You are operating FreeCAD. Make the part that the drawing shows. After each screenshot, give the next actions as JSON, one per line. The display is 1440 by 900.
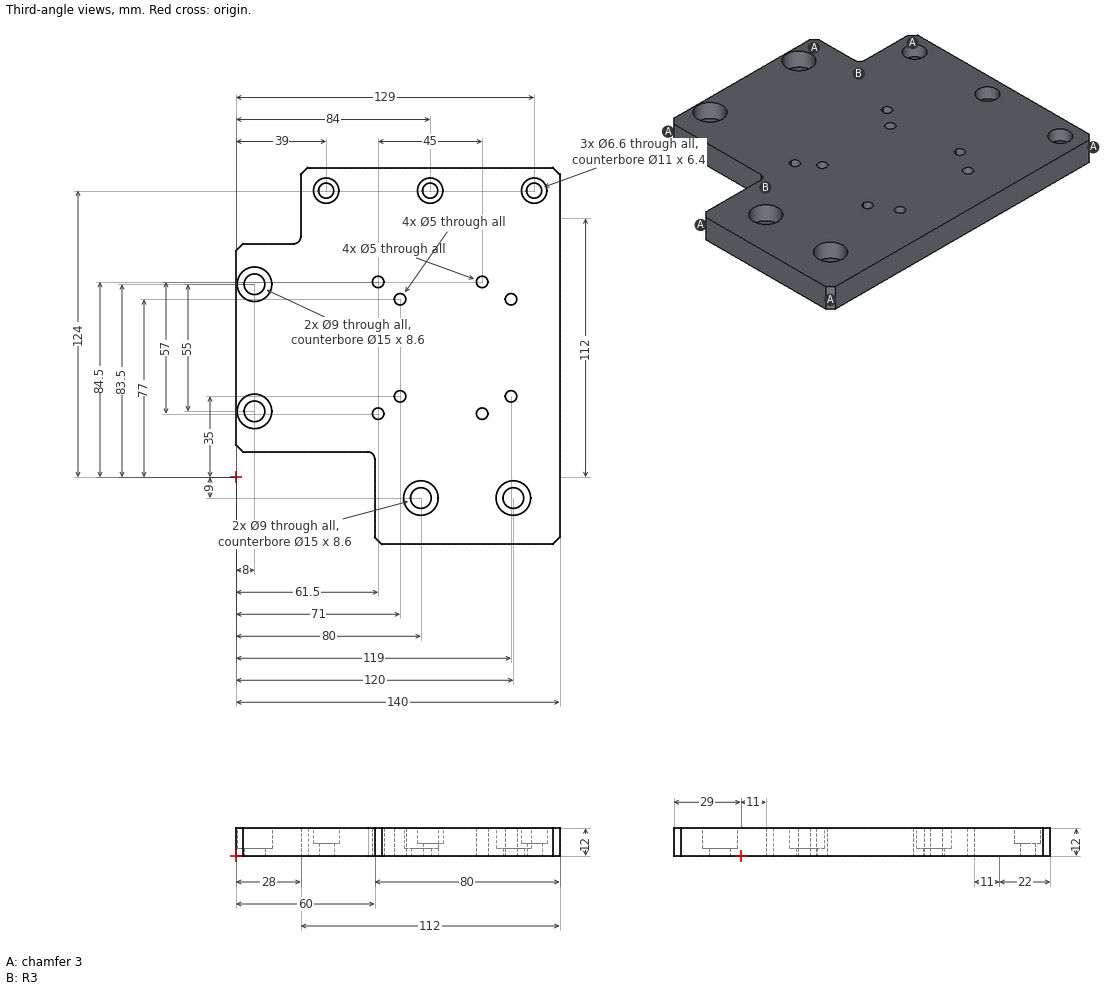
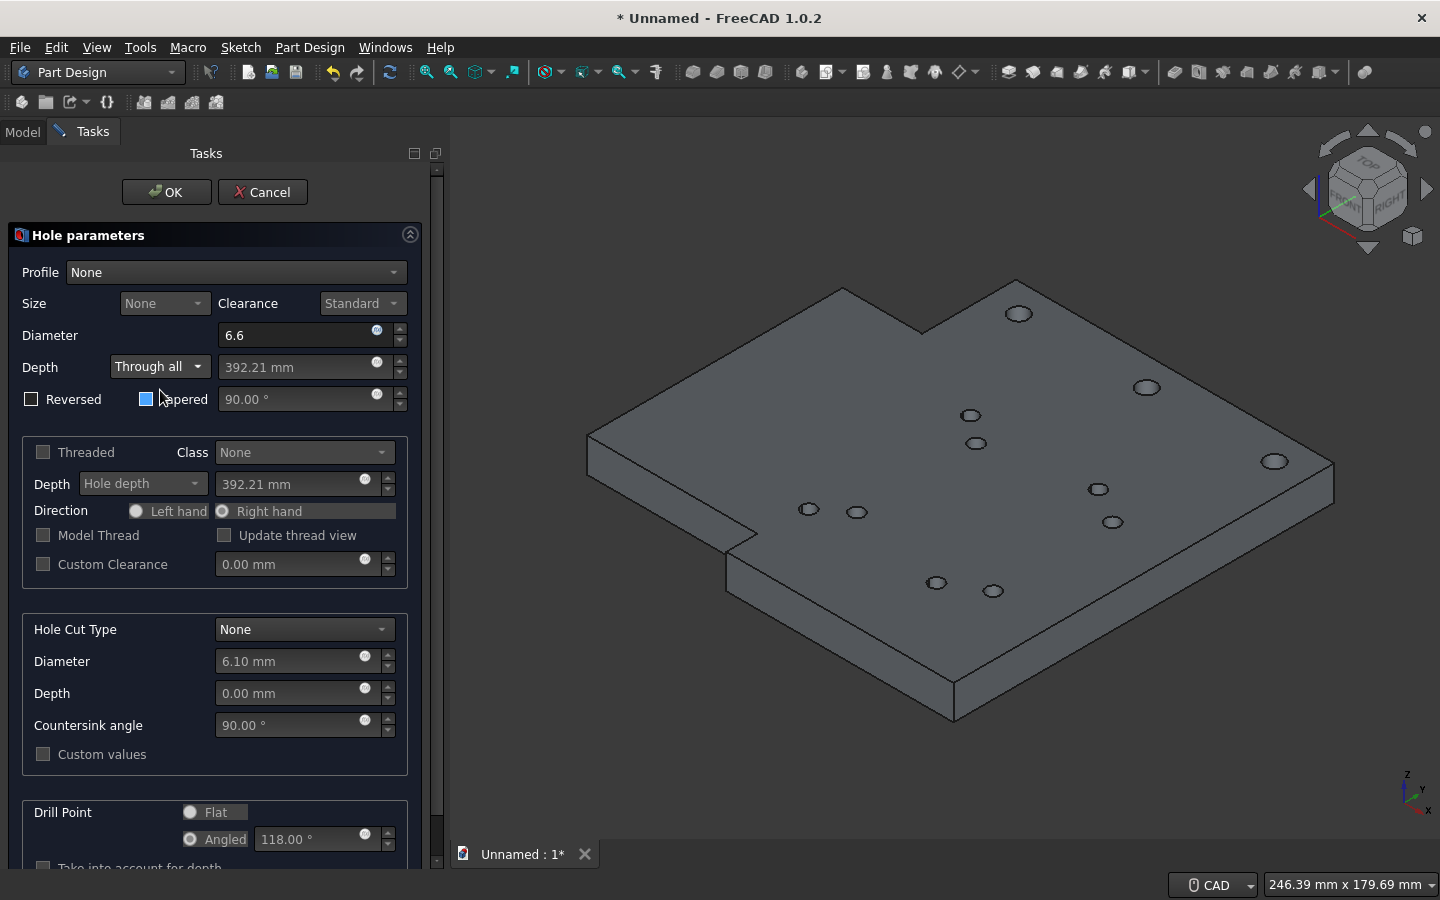
{"action": "left_click", "coordinate": [306, 630]}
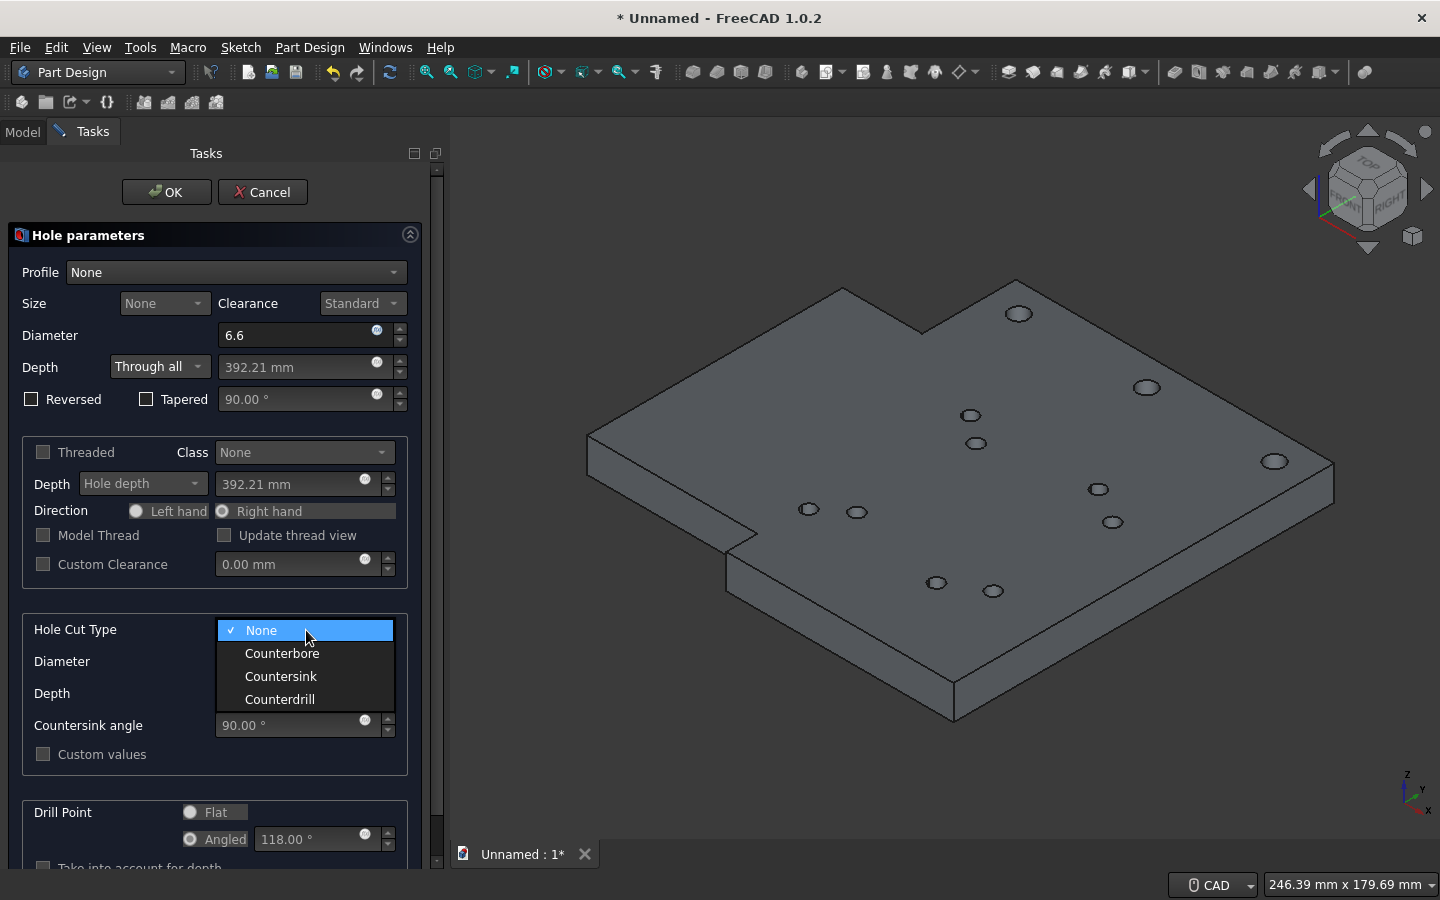
{"action": "left_click", "coordinate": [304, 654]}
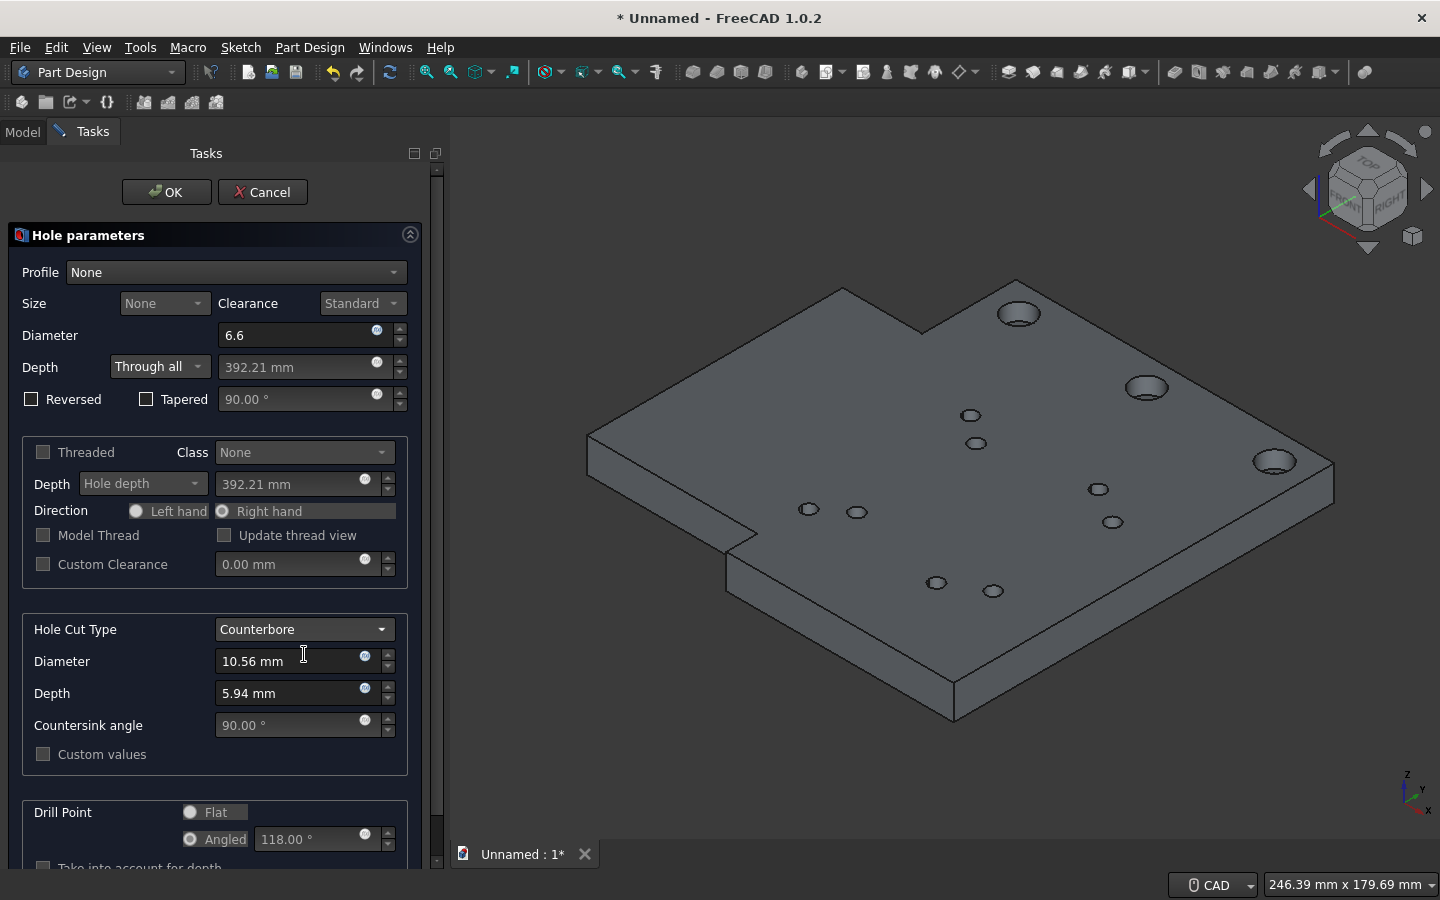
{"action": "triple_click", "coordinate": [298, 661]}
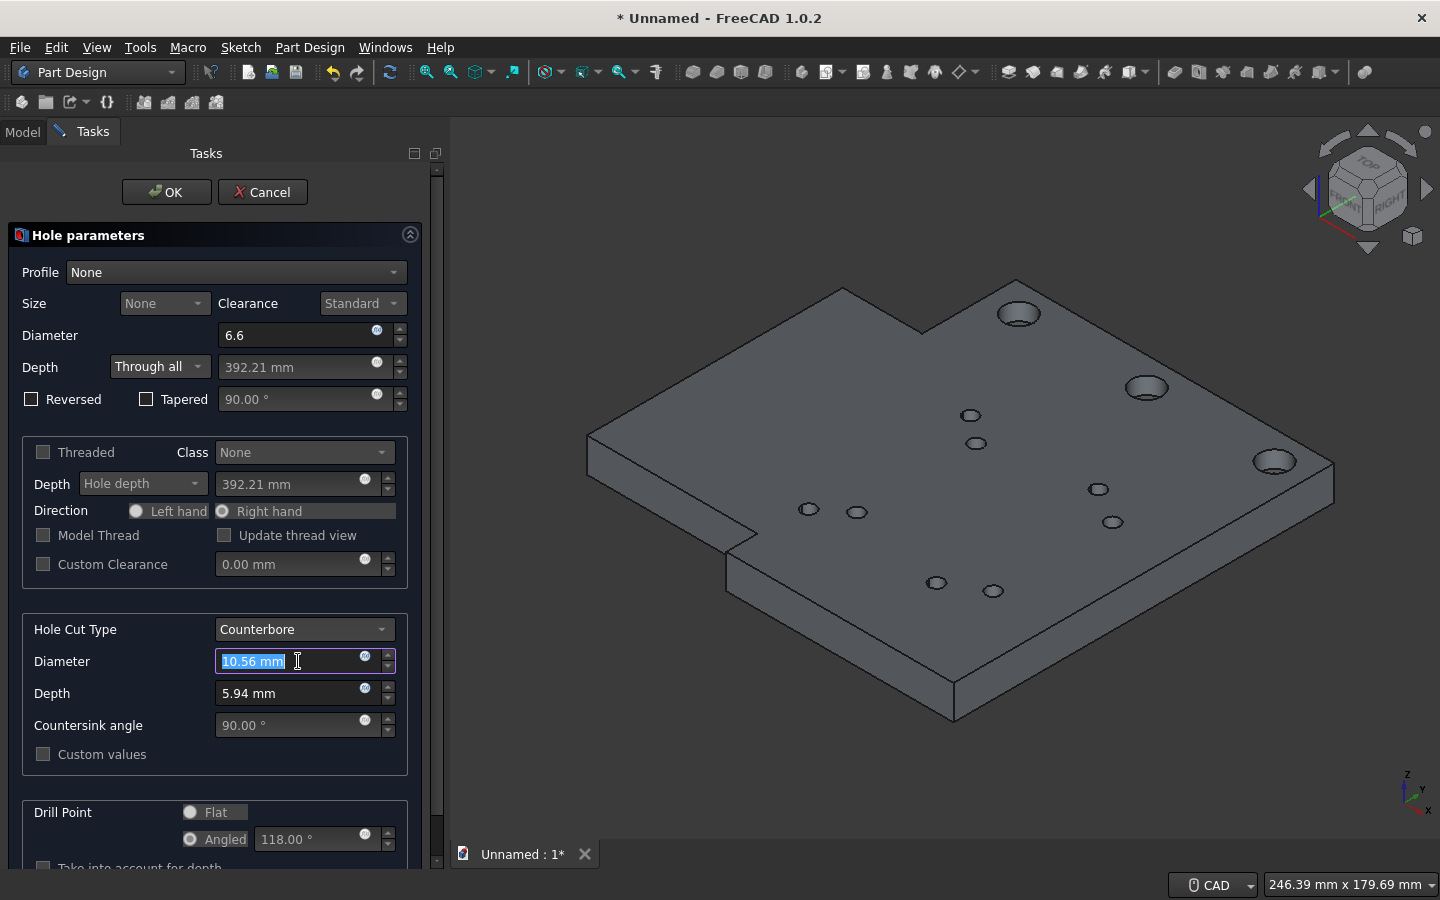
{"action": "type", "text": "11"}
{"action": "key", "text": "Tab"}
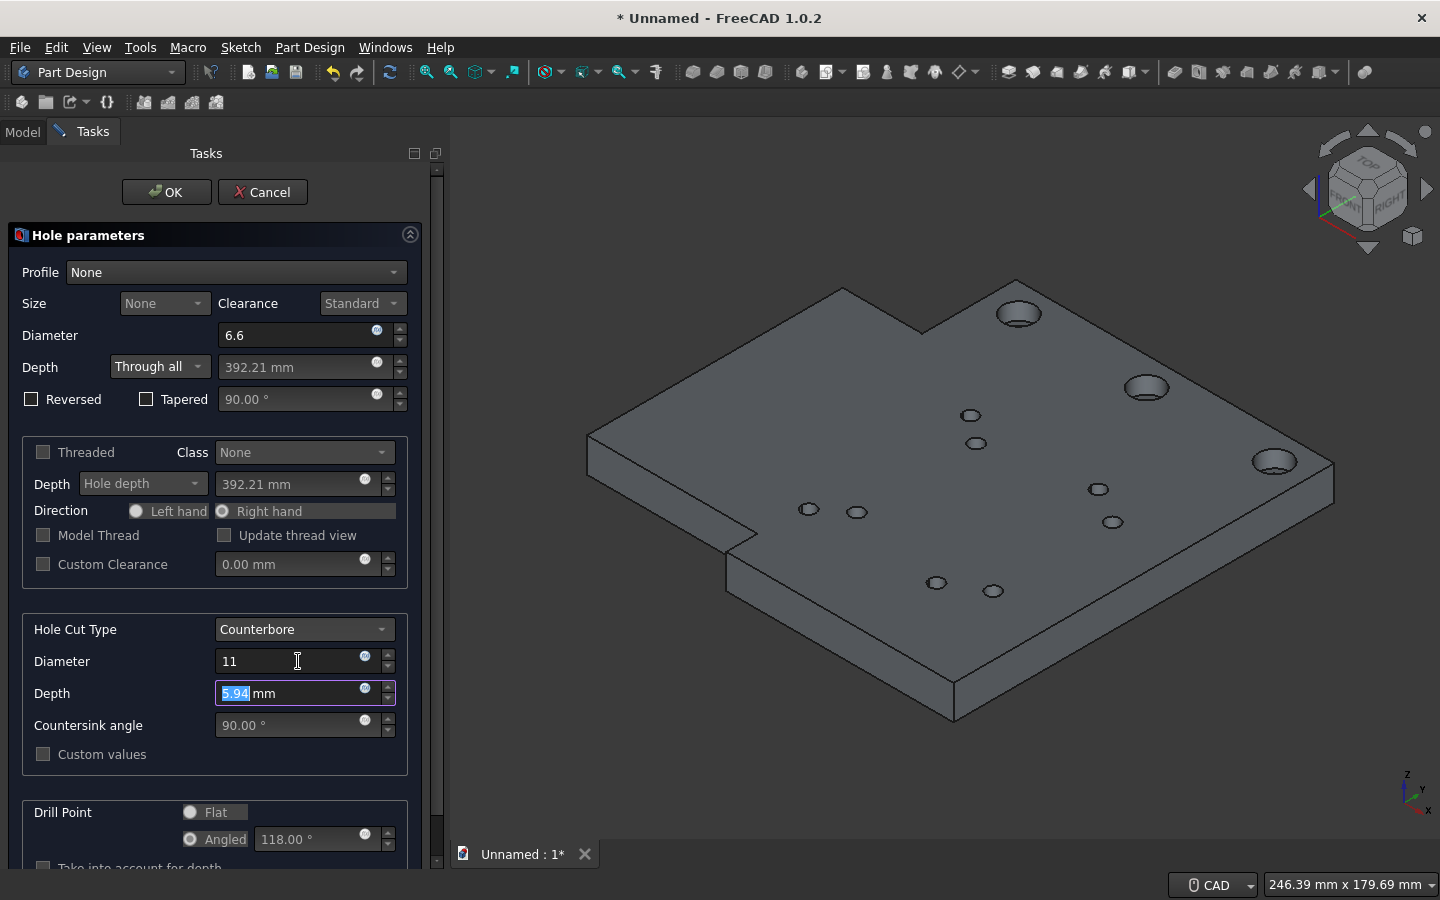
{"action": "type", "text": "6.4"}
{"action": "key", "text": "Tab"}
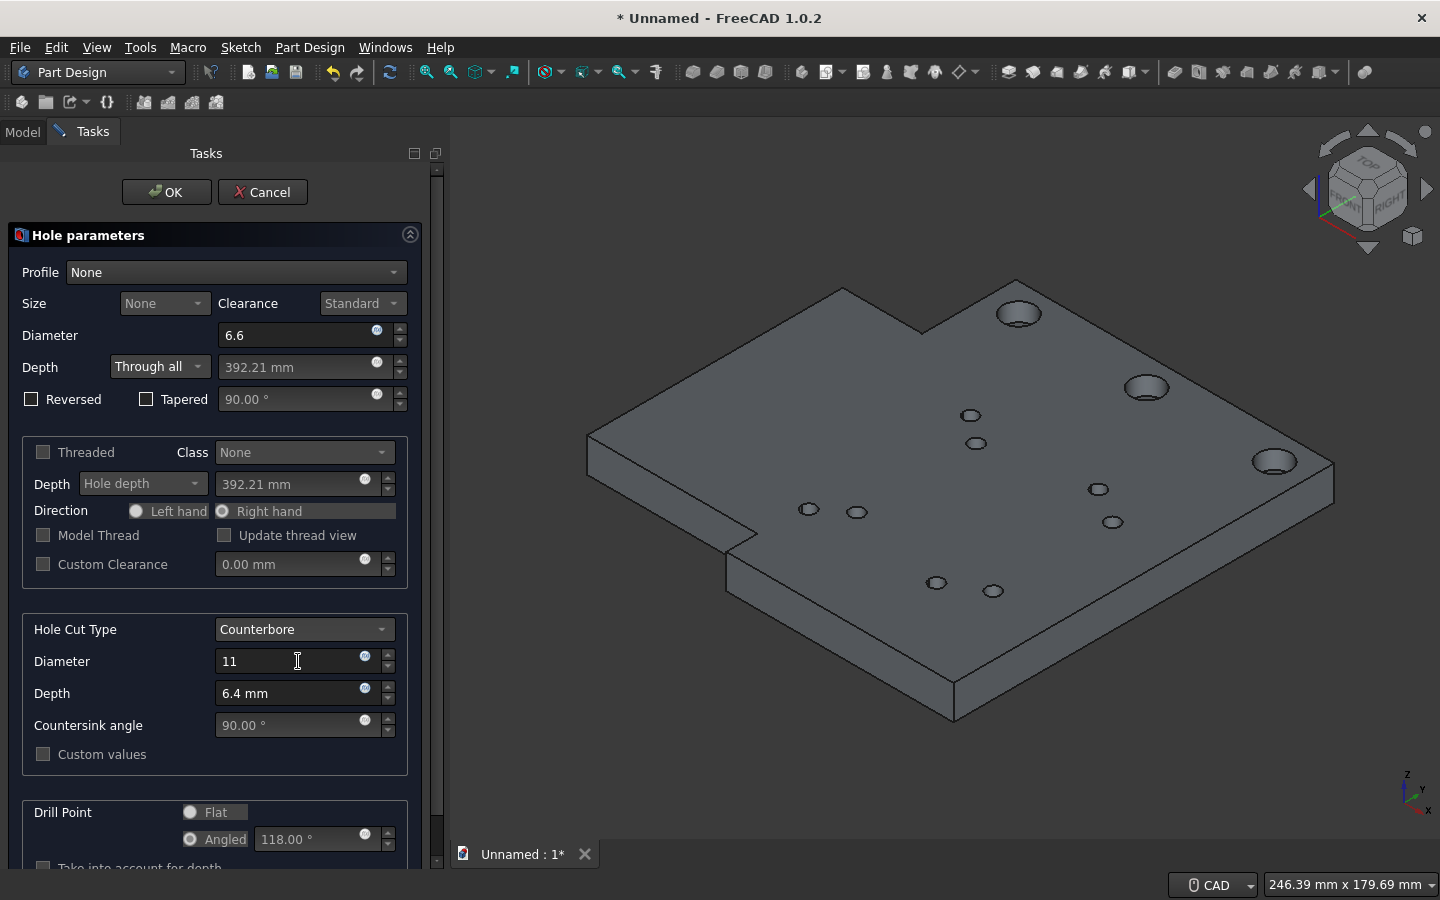
{"action": "left_click", "coordinate": [167, 192]}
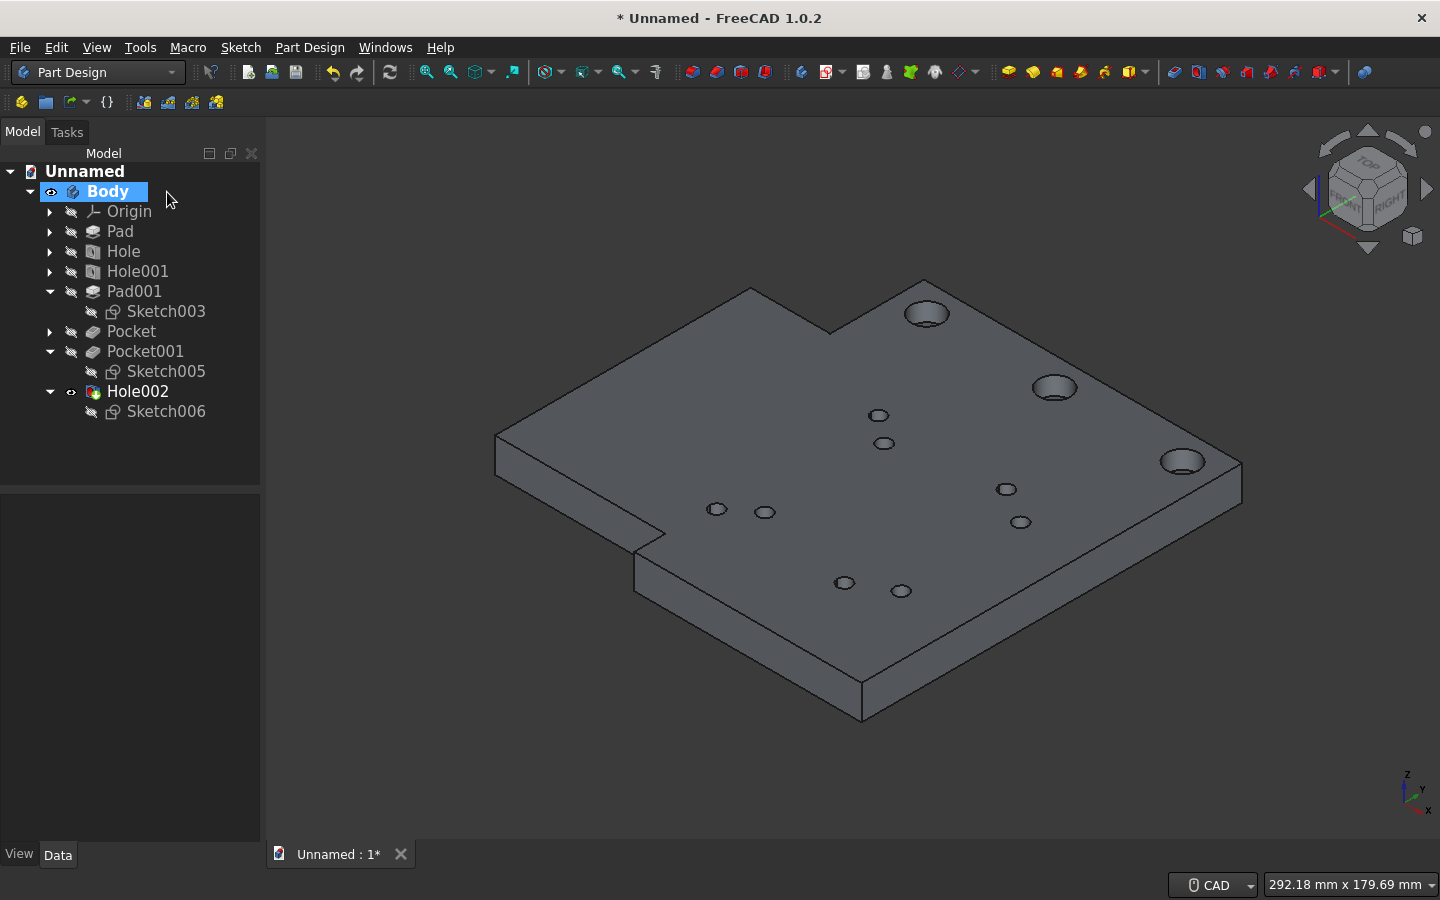
{"action": "left_click", "coordinate": [826, 72]}